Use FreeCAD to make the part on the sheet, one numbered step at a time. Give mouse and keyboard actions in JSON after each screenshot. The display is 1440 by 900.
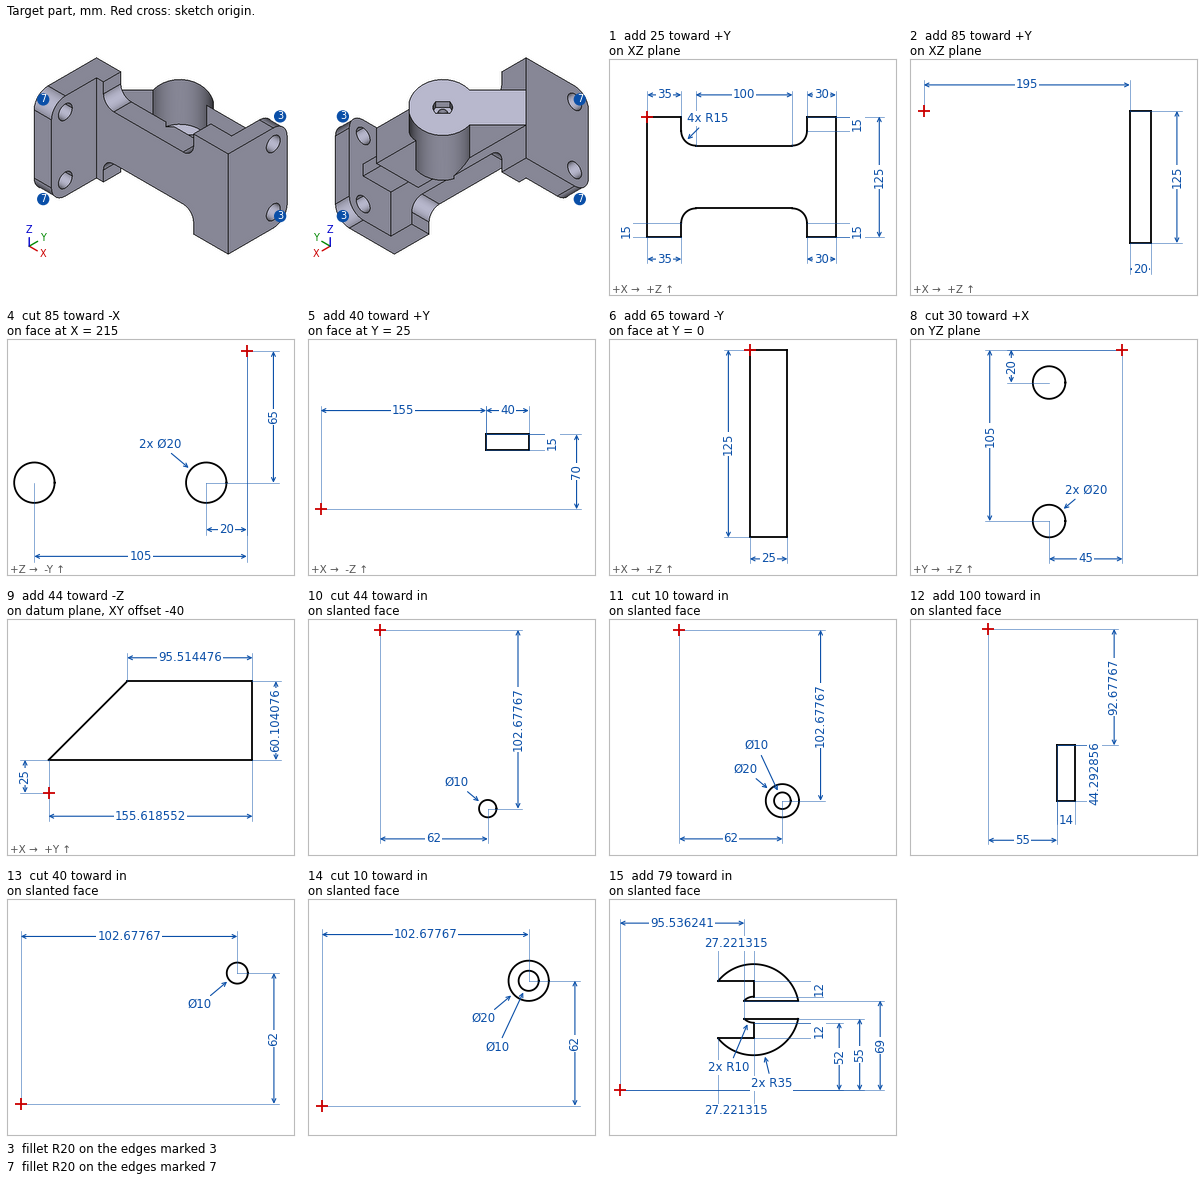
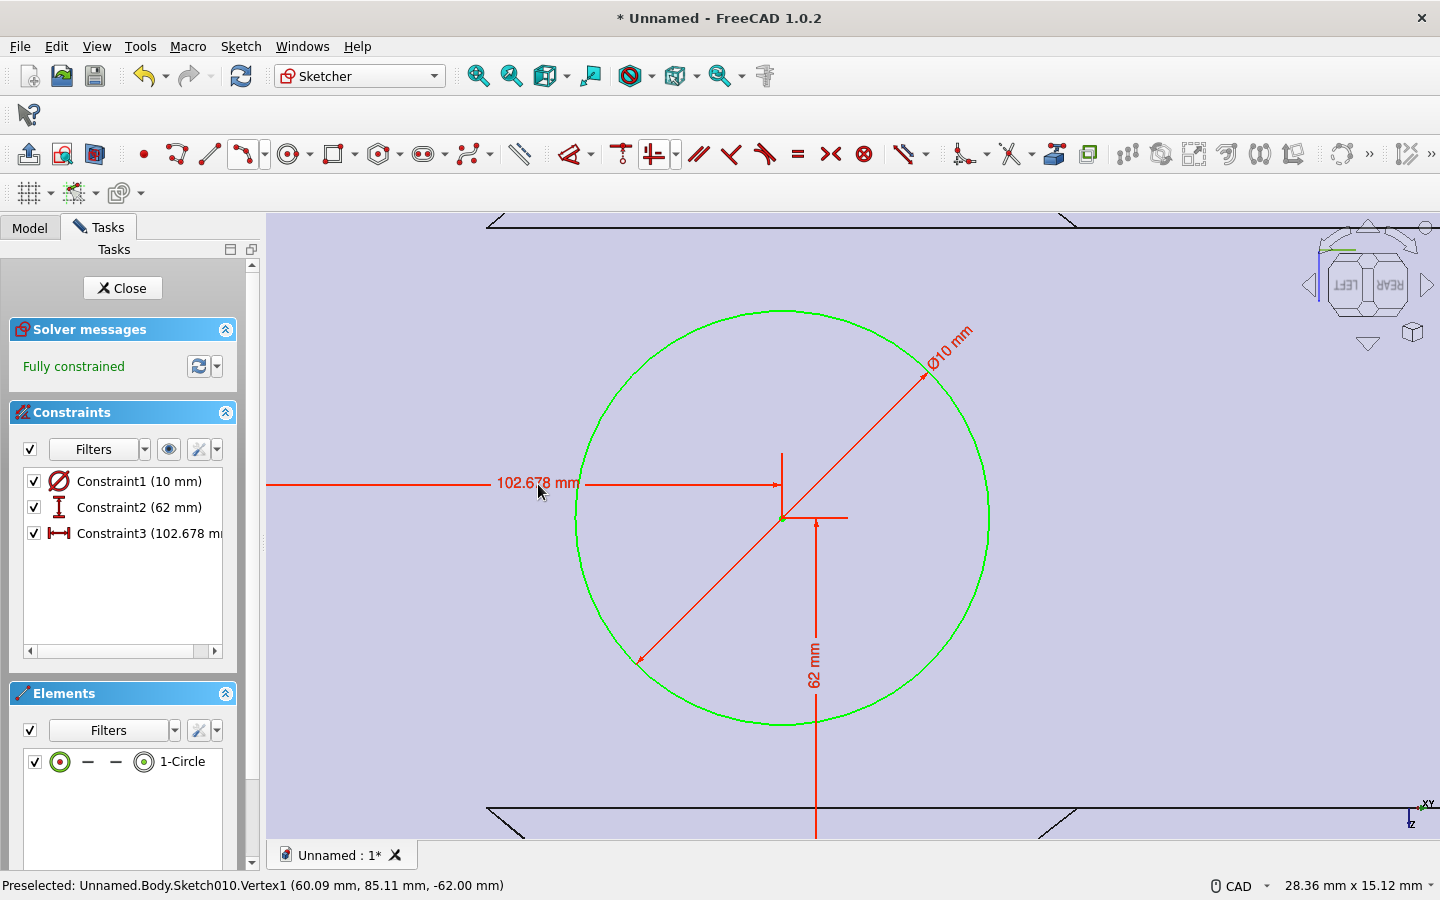
{"action": "left_click", "coordinate": [123, 288]}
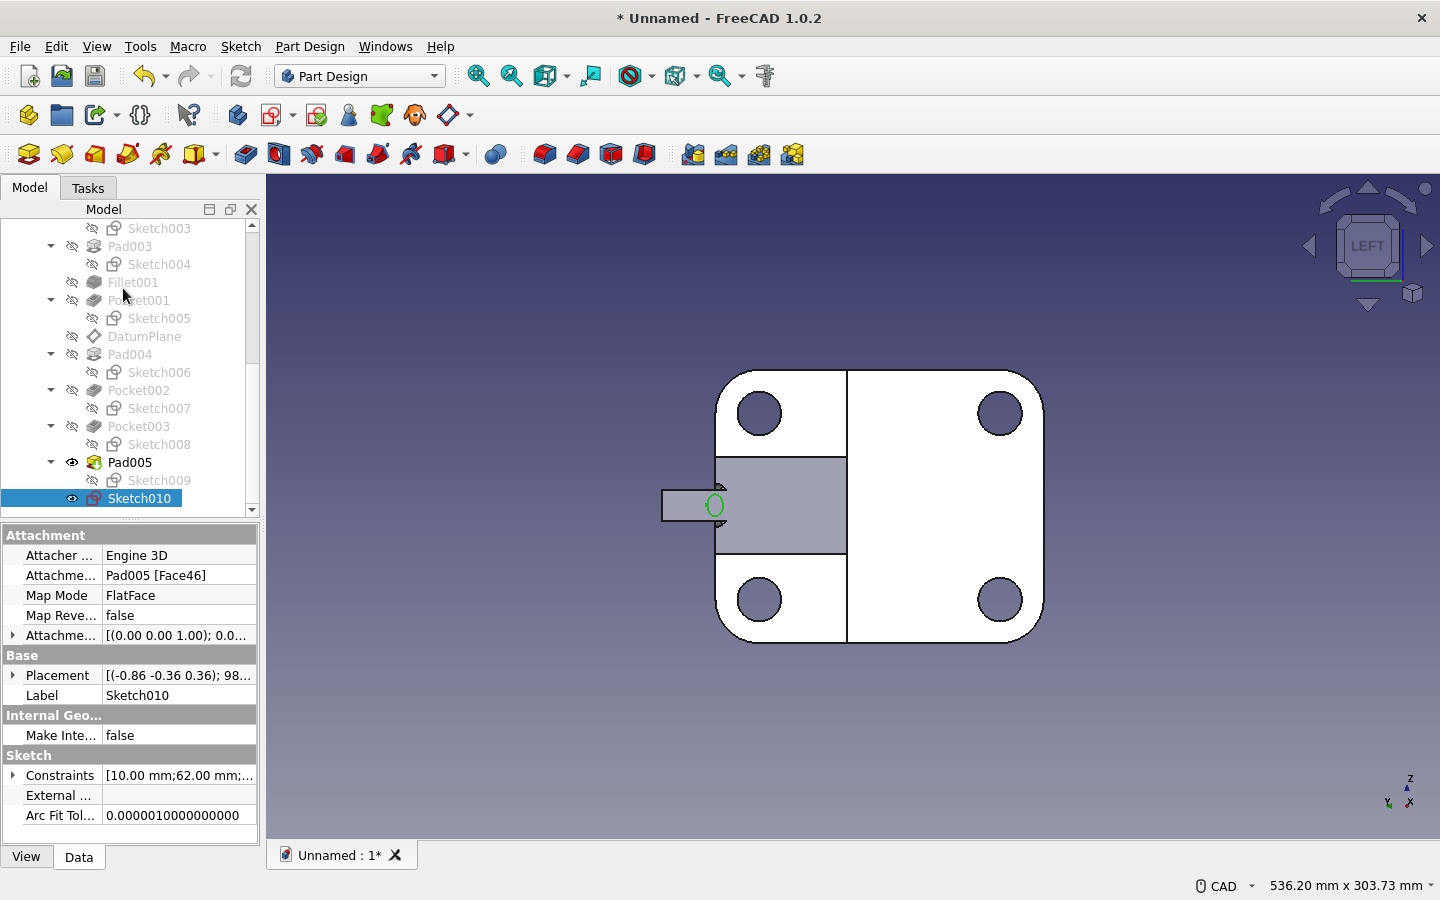
{"action": "left_click", "coordinate": [246, 154]}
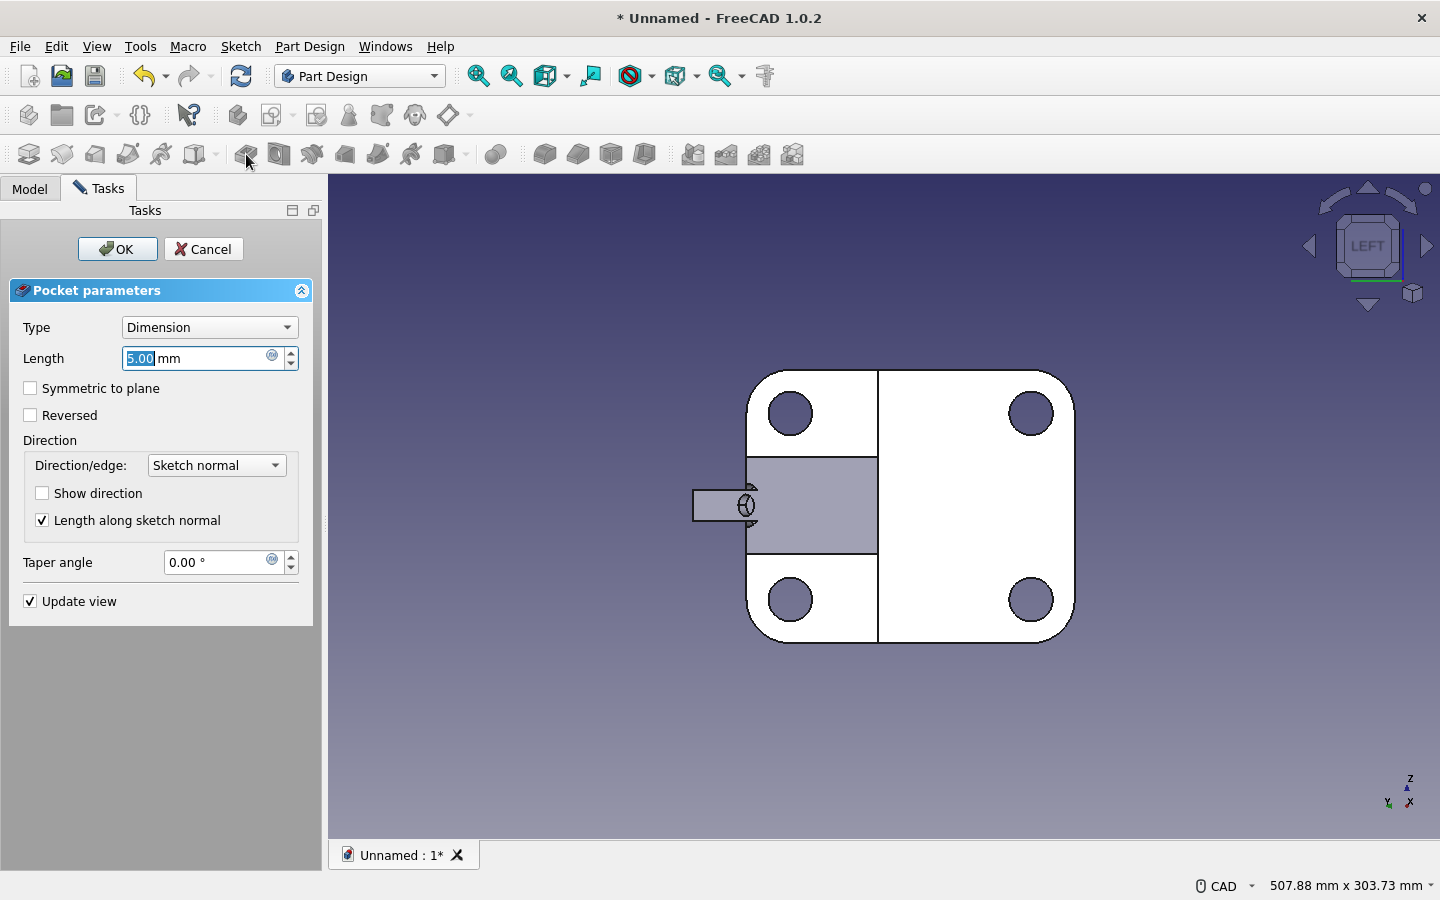
{"action": "type", "text": "40"}
{"action": "key", "text": "Tab"}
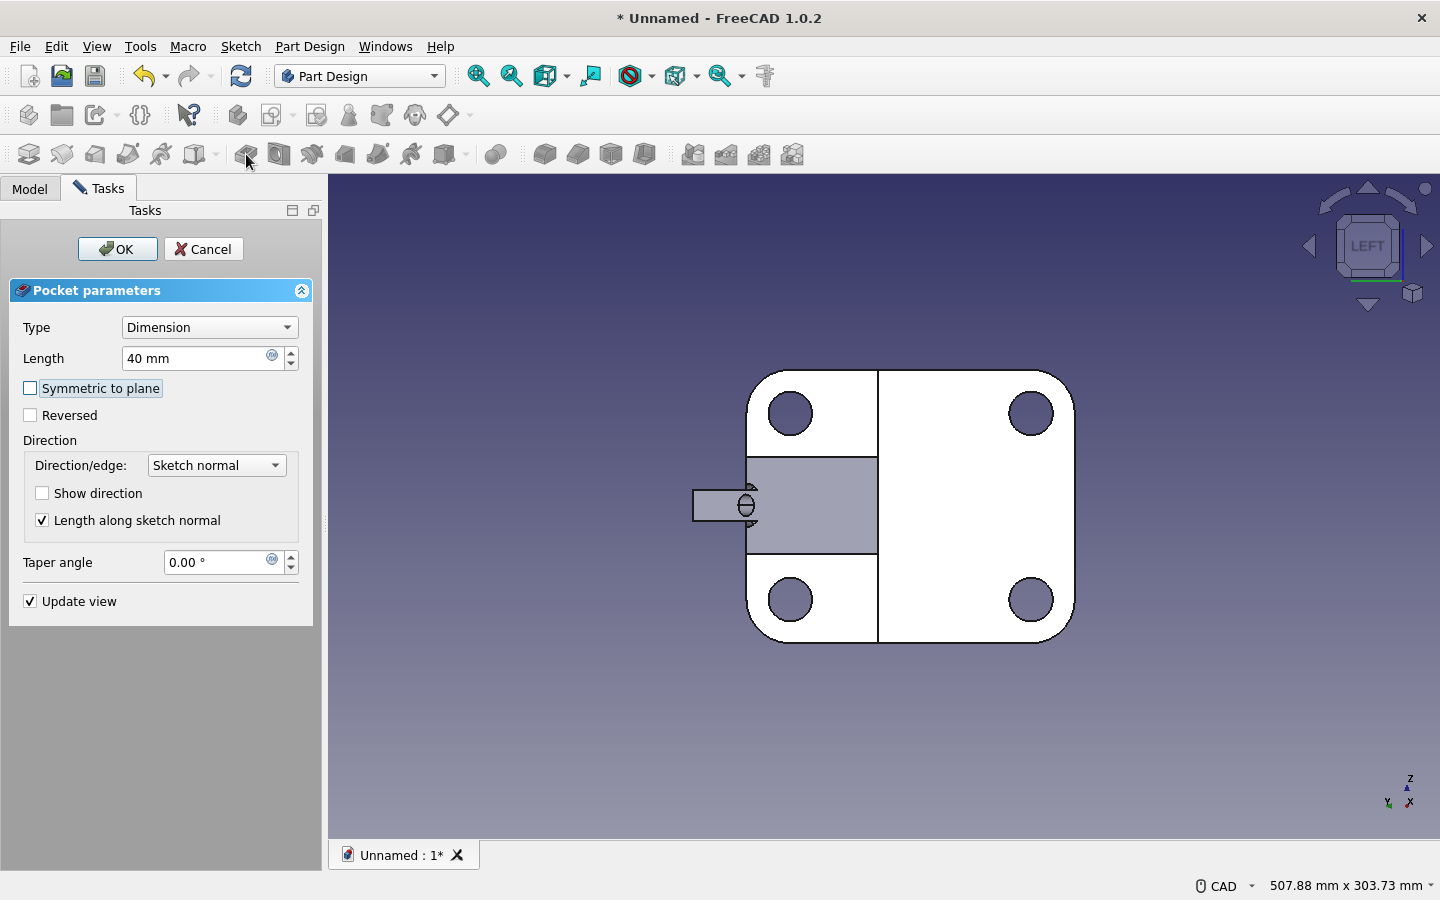
{"action": "left_click", "coordinate": [118, 249]}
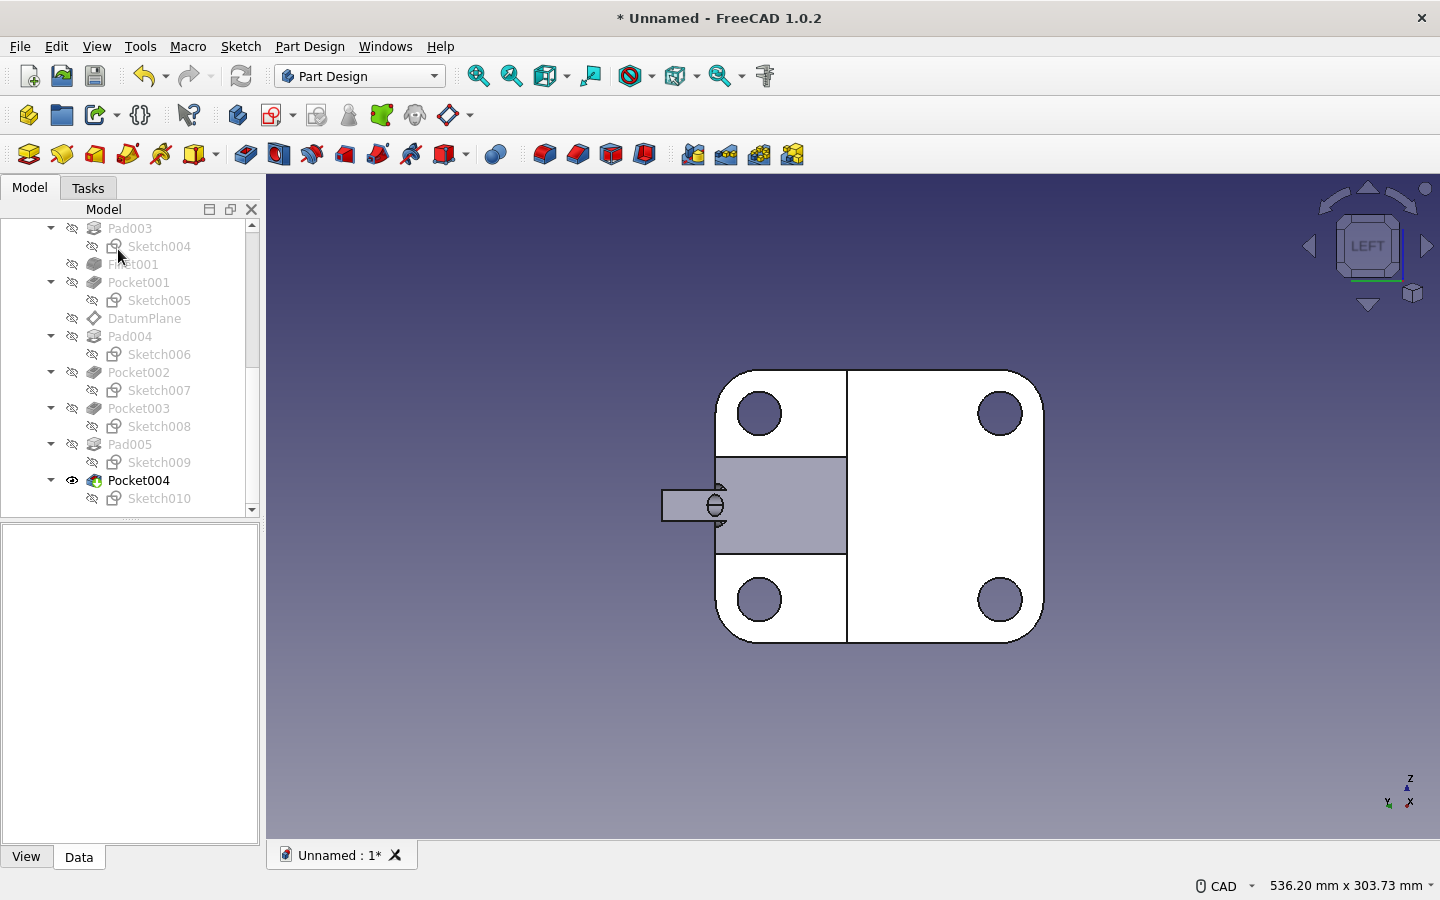
{"action": "left_click", "coordinate": [479, 76]}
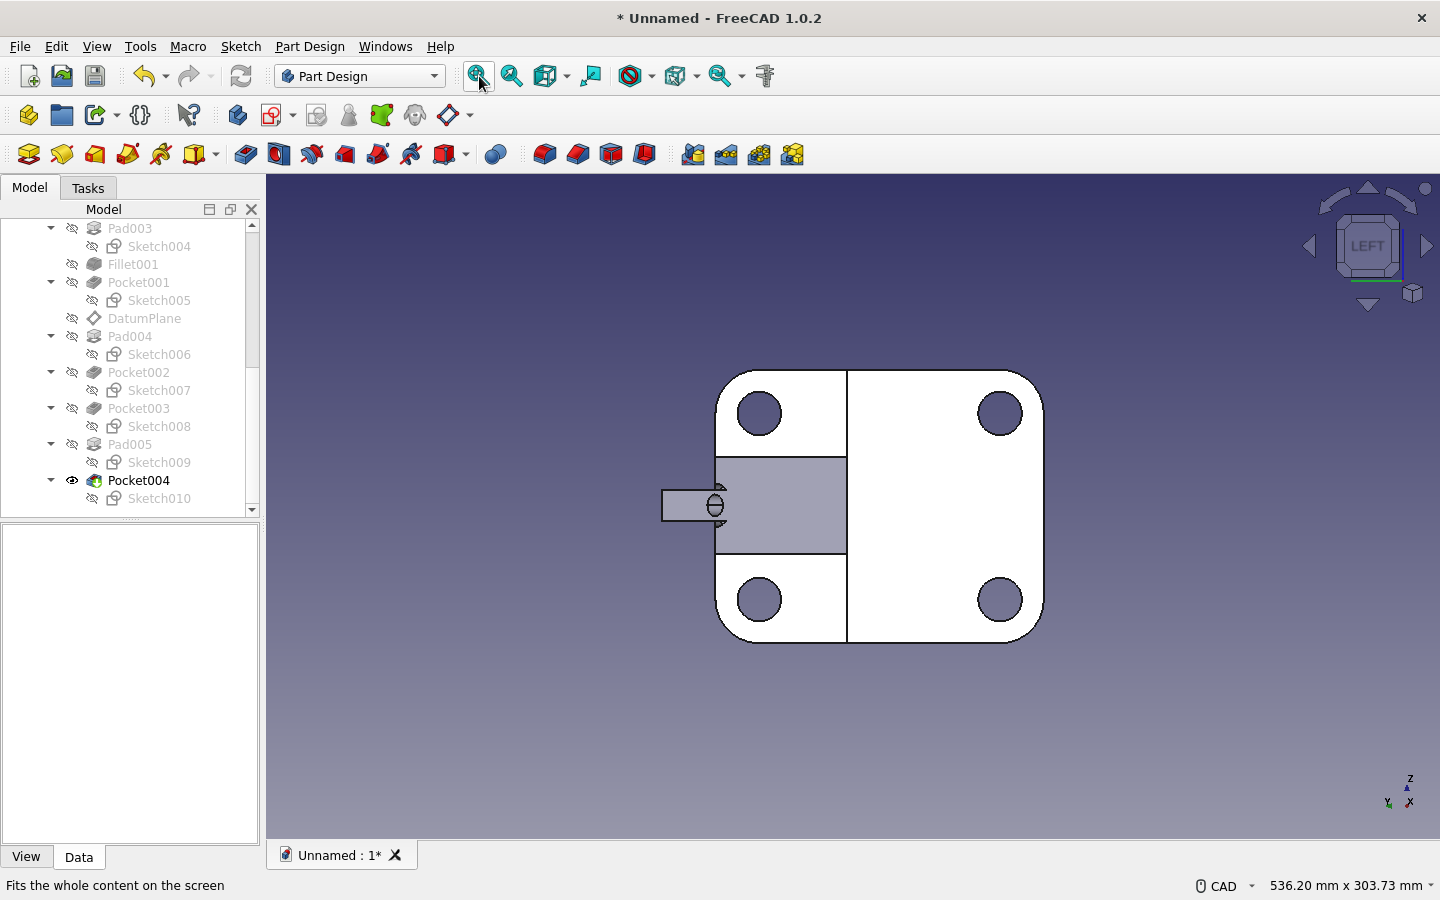
{"action": "left_click", "coordinate": [781, 504]}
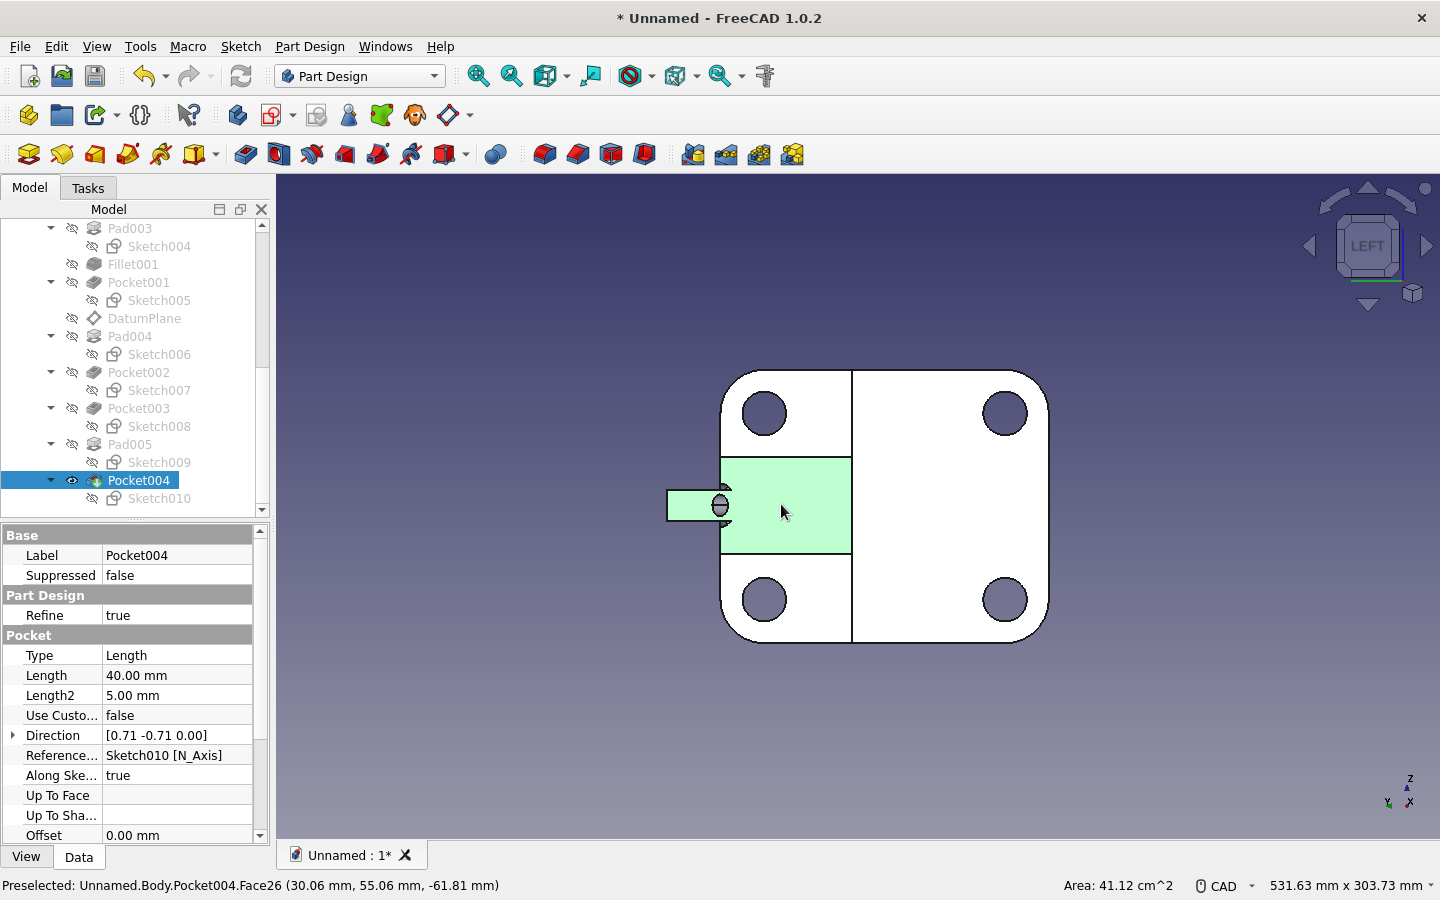
{"action": "left_click", "coordinate": [270, 116]}